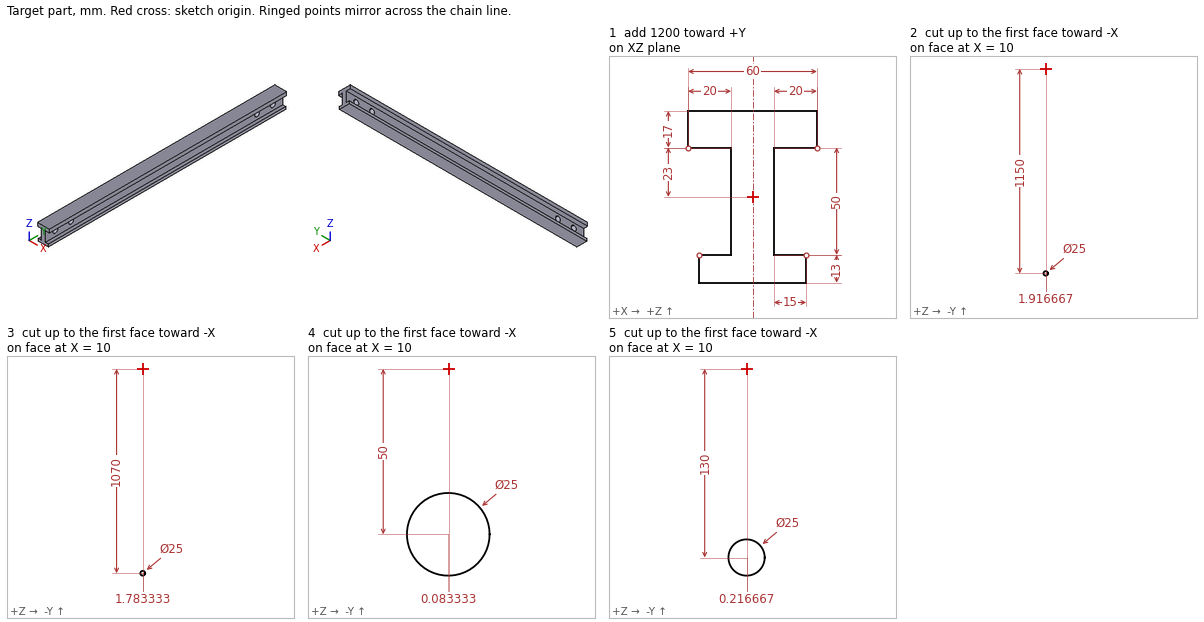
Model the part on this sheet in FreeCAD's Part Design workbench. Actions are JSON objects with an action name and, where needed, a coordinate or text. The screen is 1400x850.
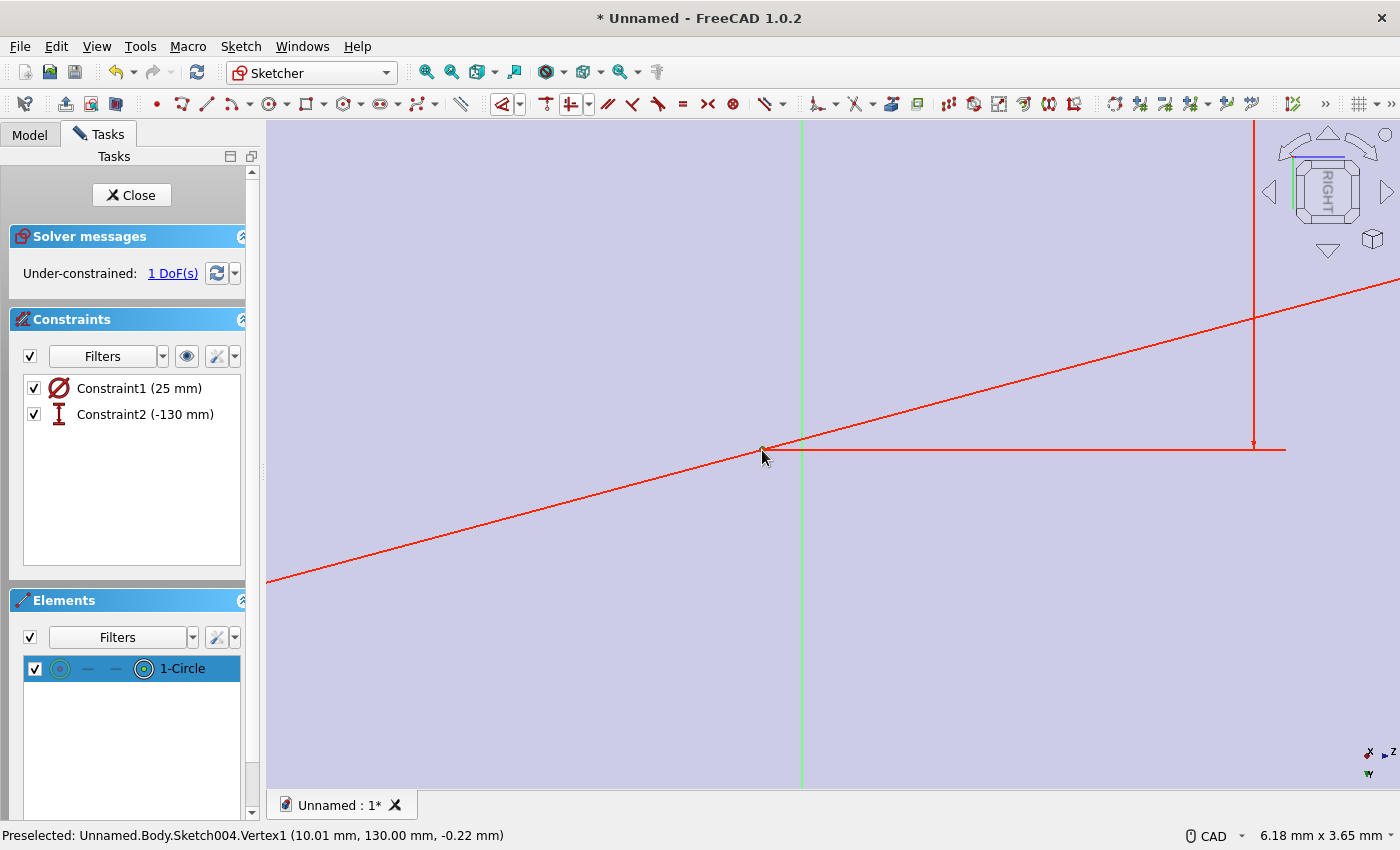
{"action": "key", "text": "l"}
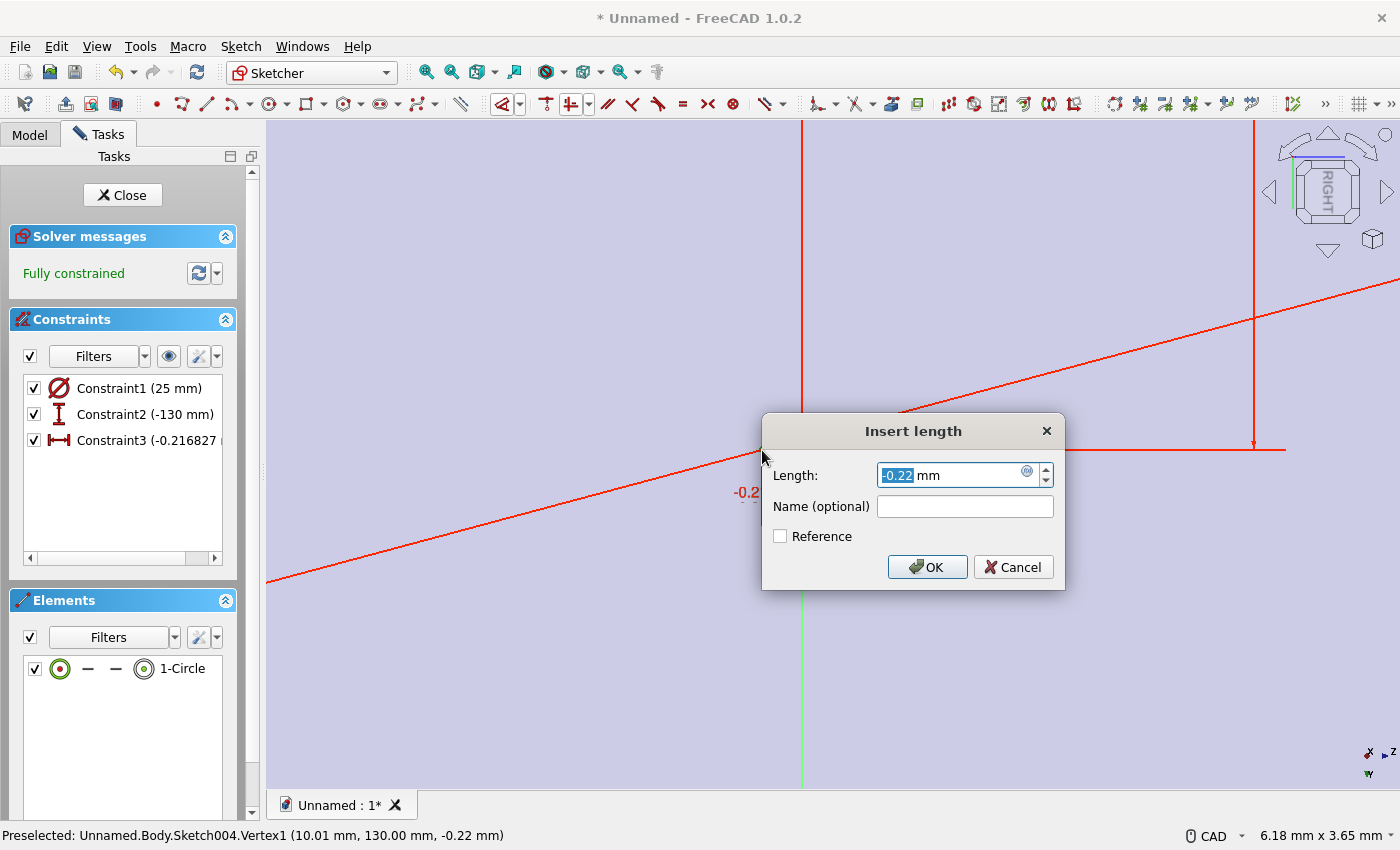
{"action": "type", "text": "-0.216667"}
{"action": "key", "text": "Return"}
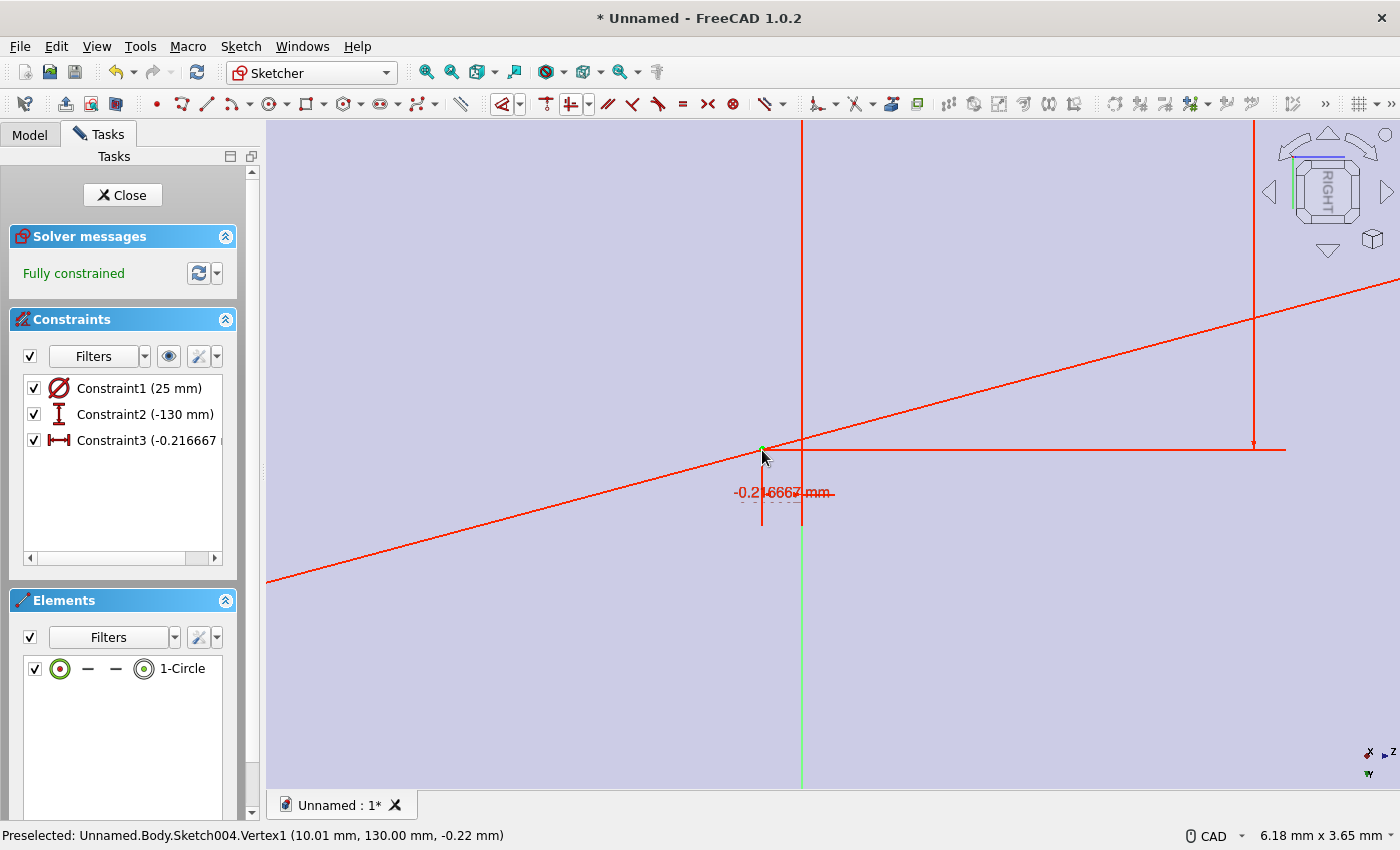
{"action": "left_click", "coordinate": [123, 195]}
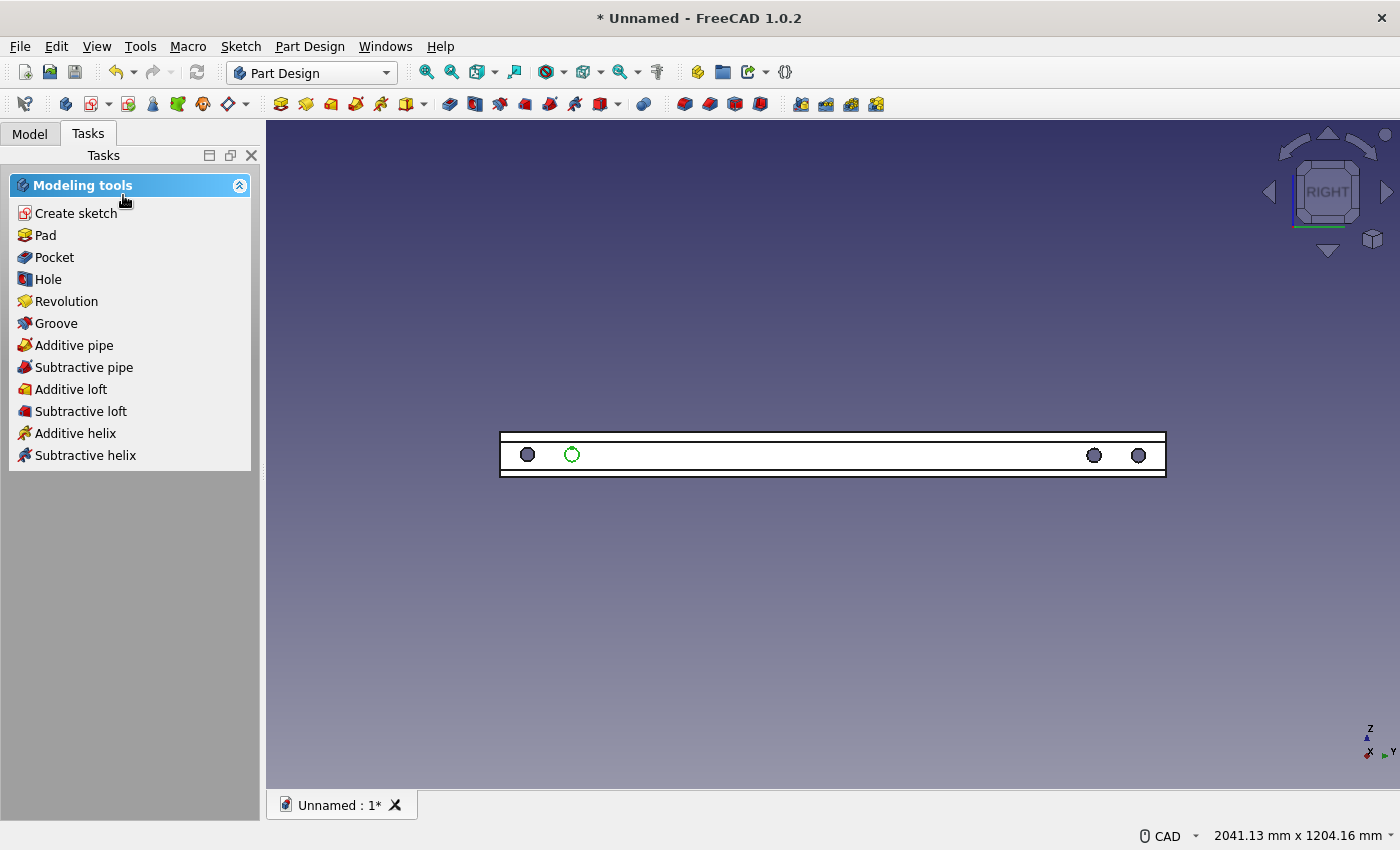
{"action": "left_click", "coordinate": [450, 104]}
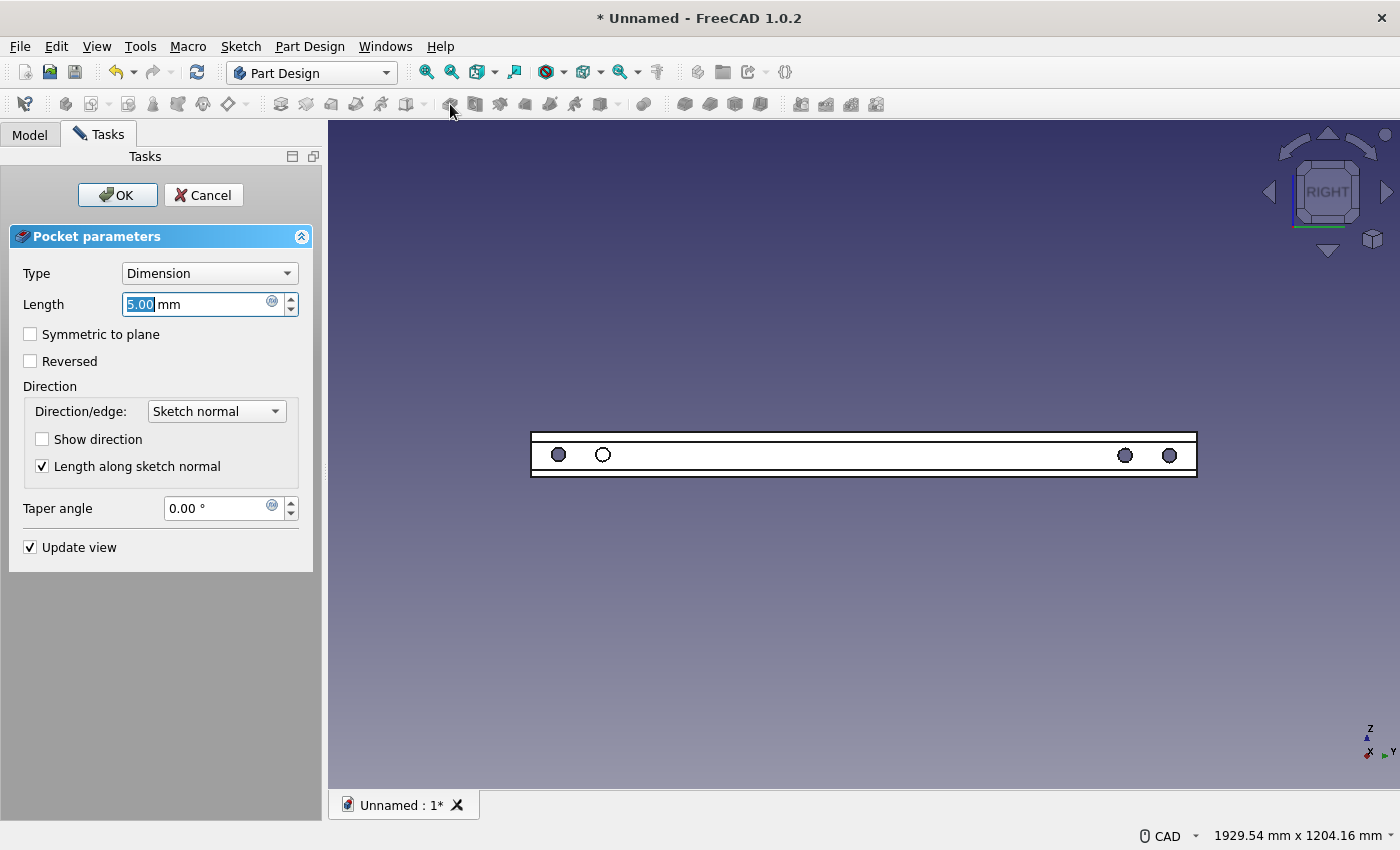
{"action": "left_click", "coordinate": [210, 274]}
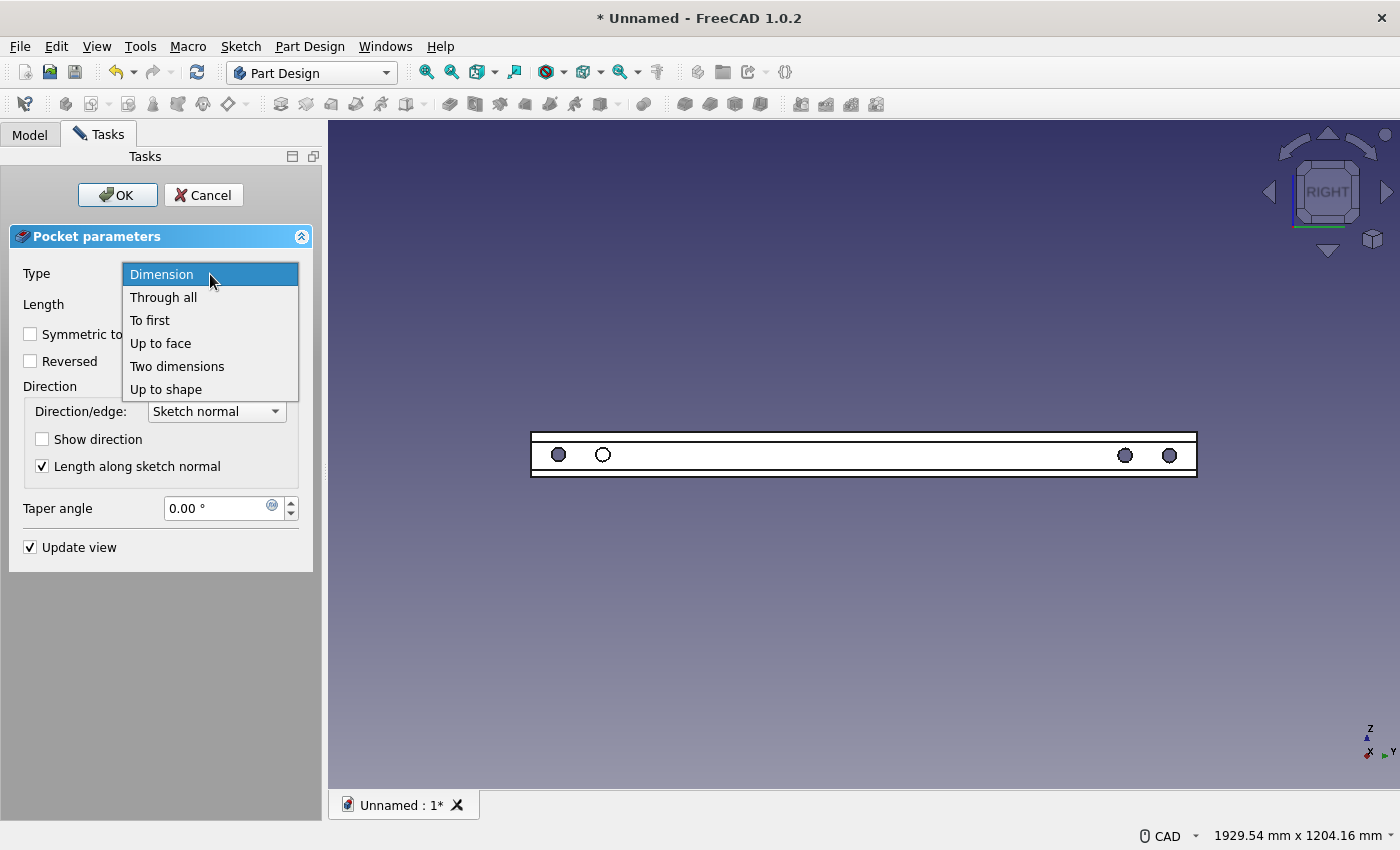
{"action": "left_click", "coordinate": [208, 320]}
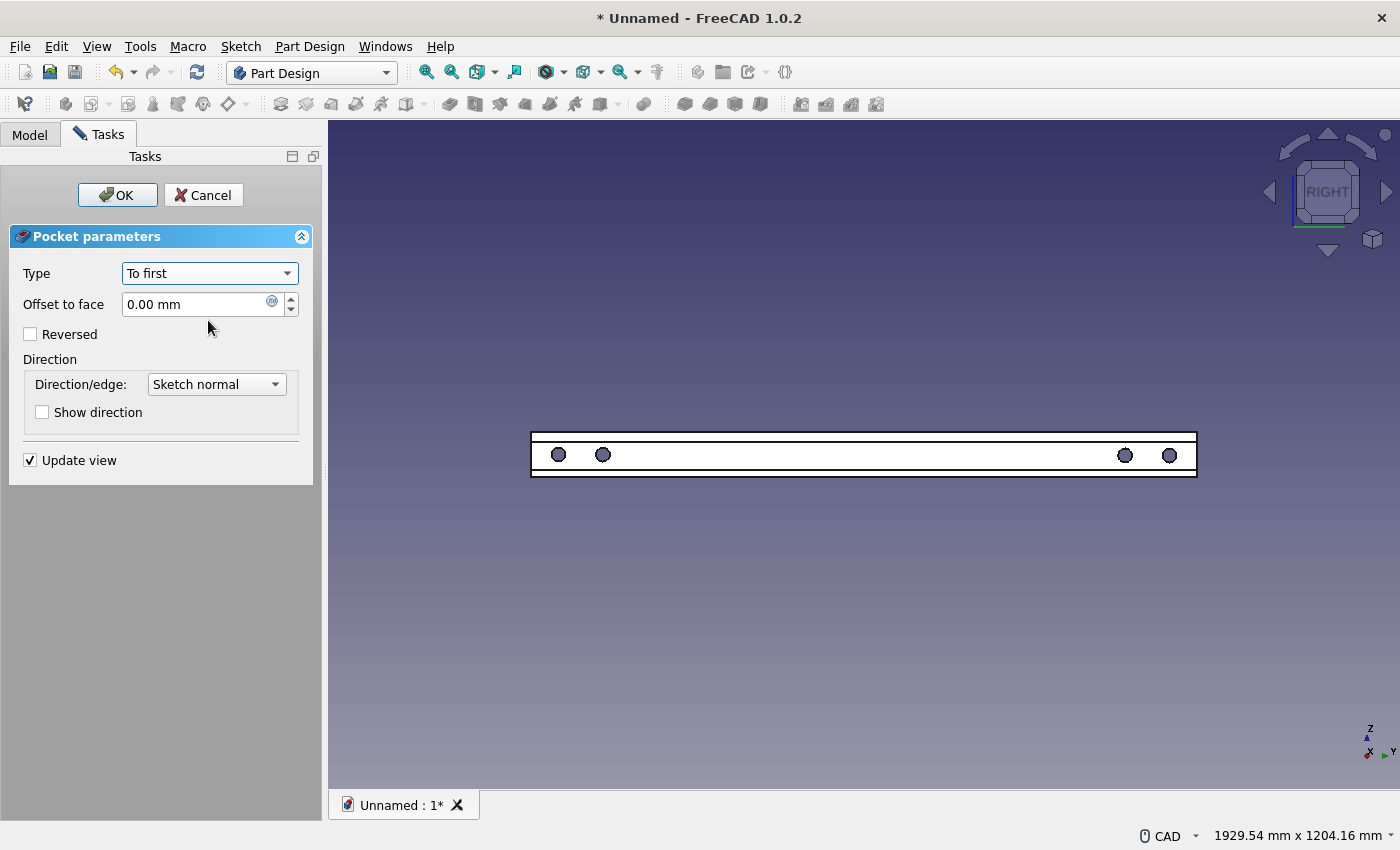
{"action": "left_click", "coordinate": [118, 195]}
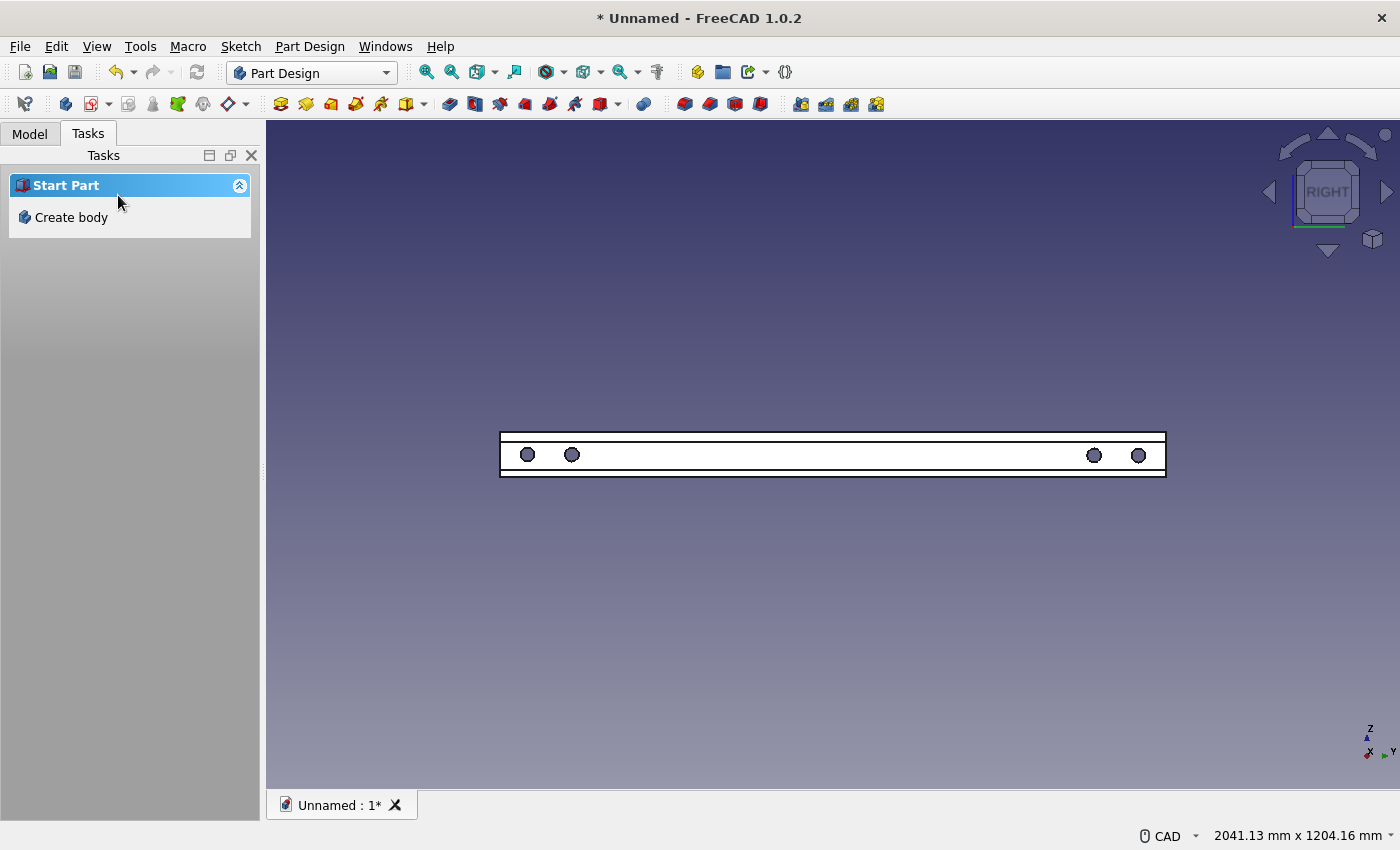
{"action": "key", "text": "0"}